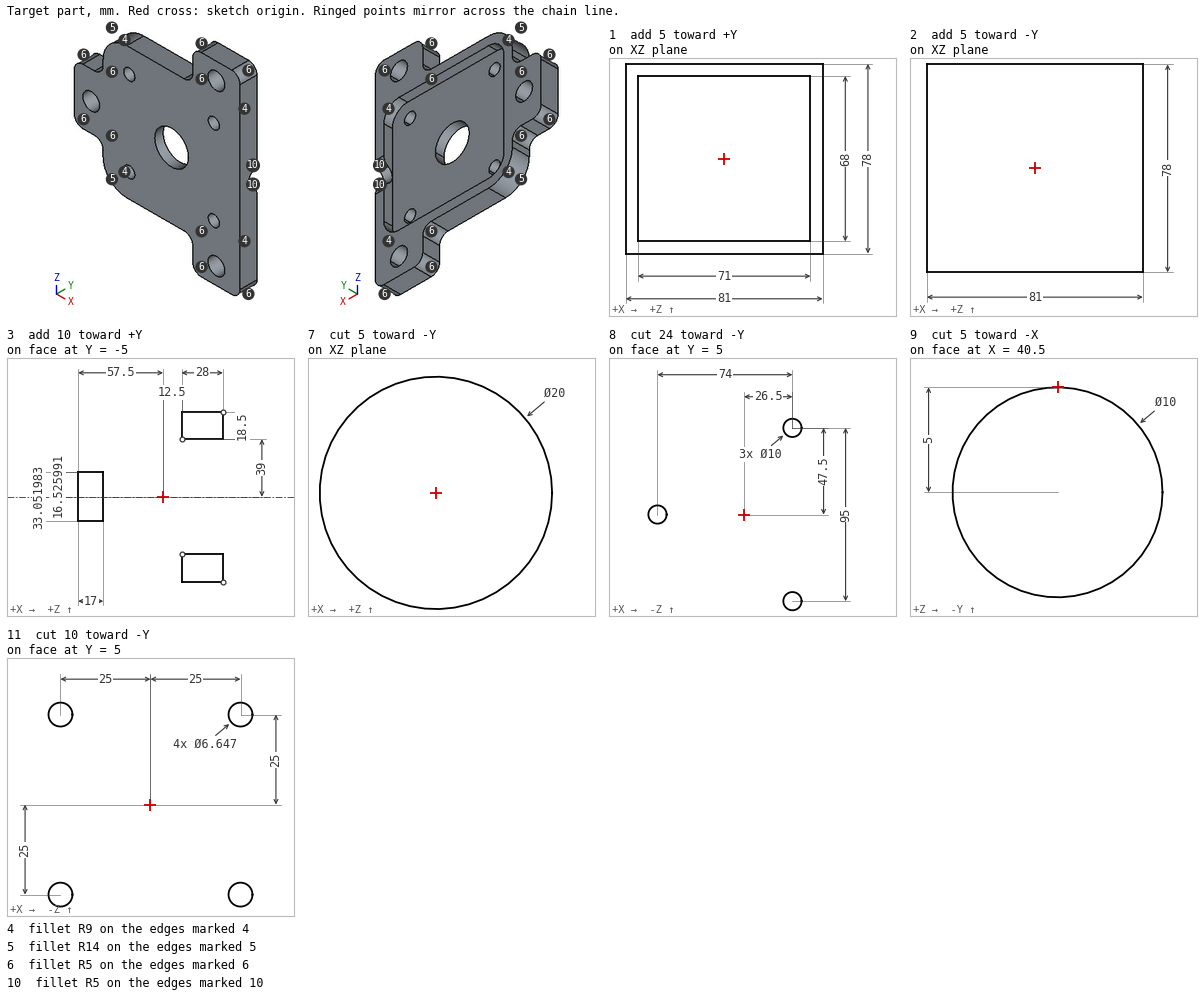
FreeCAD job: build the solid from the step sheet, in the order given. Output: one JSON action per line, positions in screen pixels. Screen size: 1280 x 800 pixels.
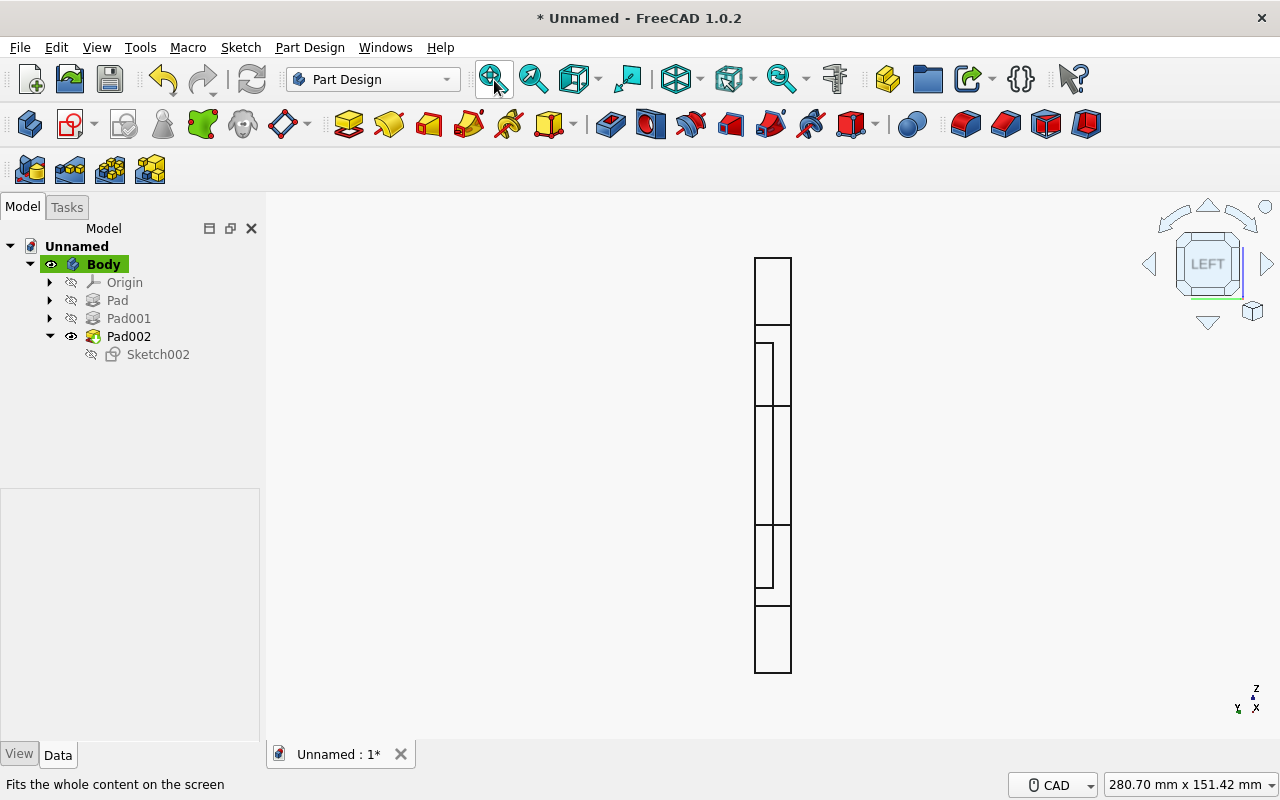
{"action": "key", "text": "0"}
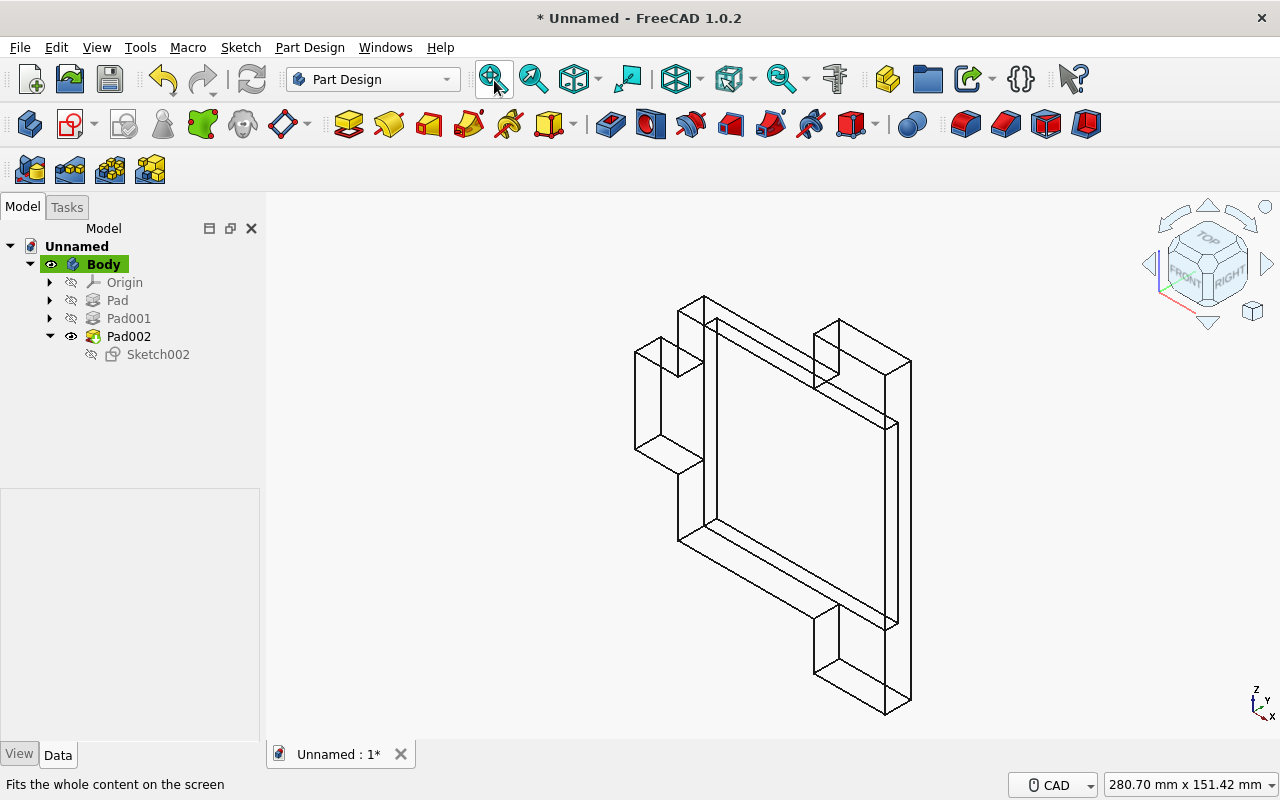
{"action": "left_click", "coordinate": [892, 425]}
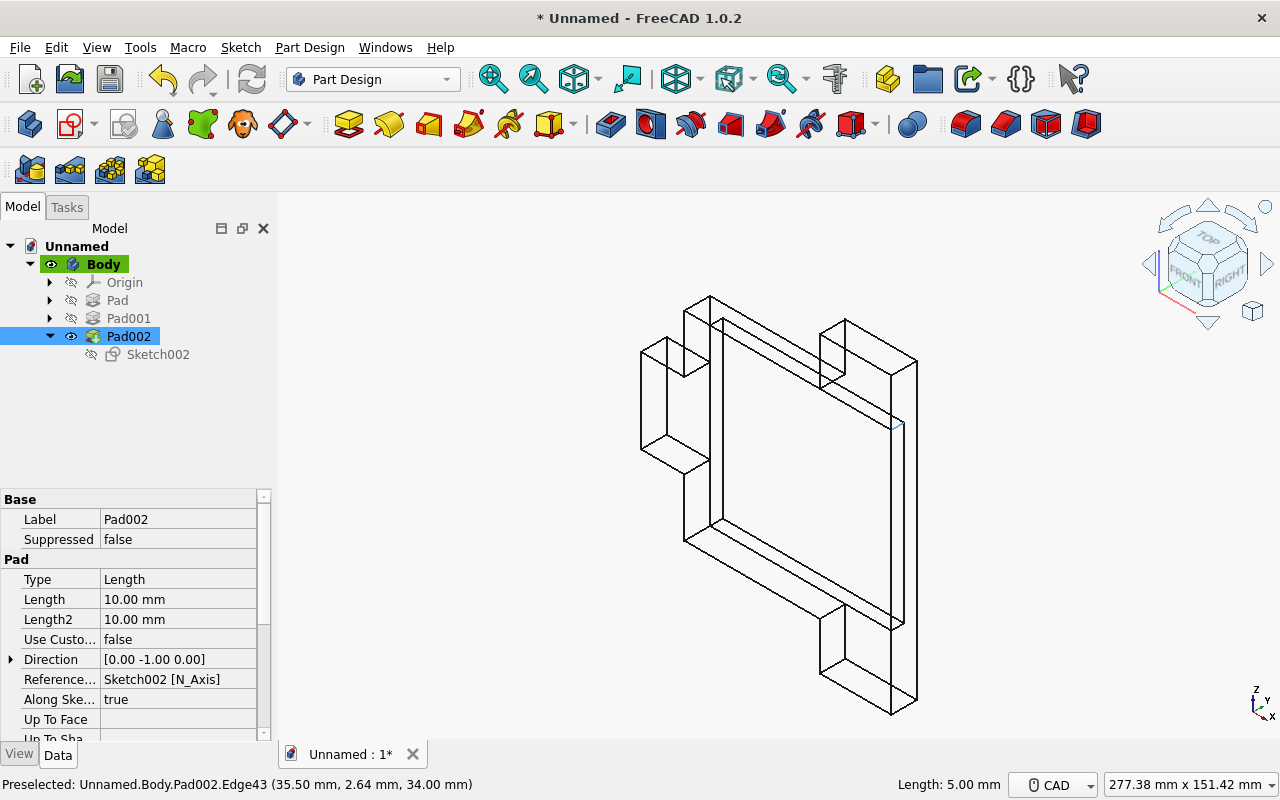
{"action": "left_click", "coordinate": [898, 626], "text": "ctrl"}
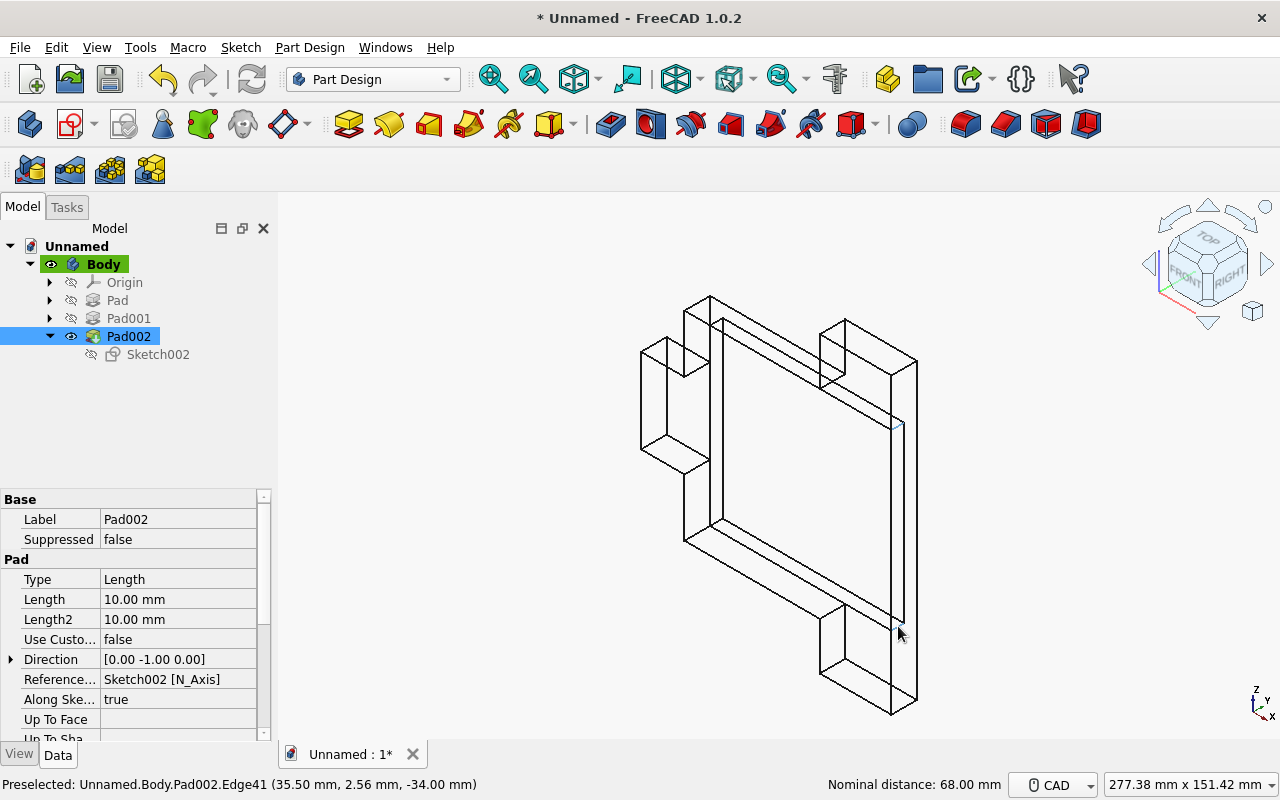
{"action": "left_click", "coordinate": [718, 521], "text": "ctrl"}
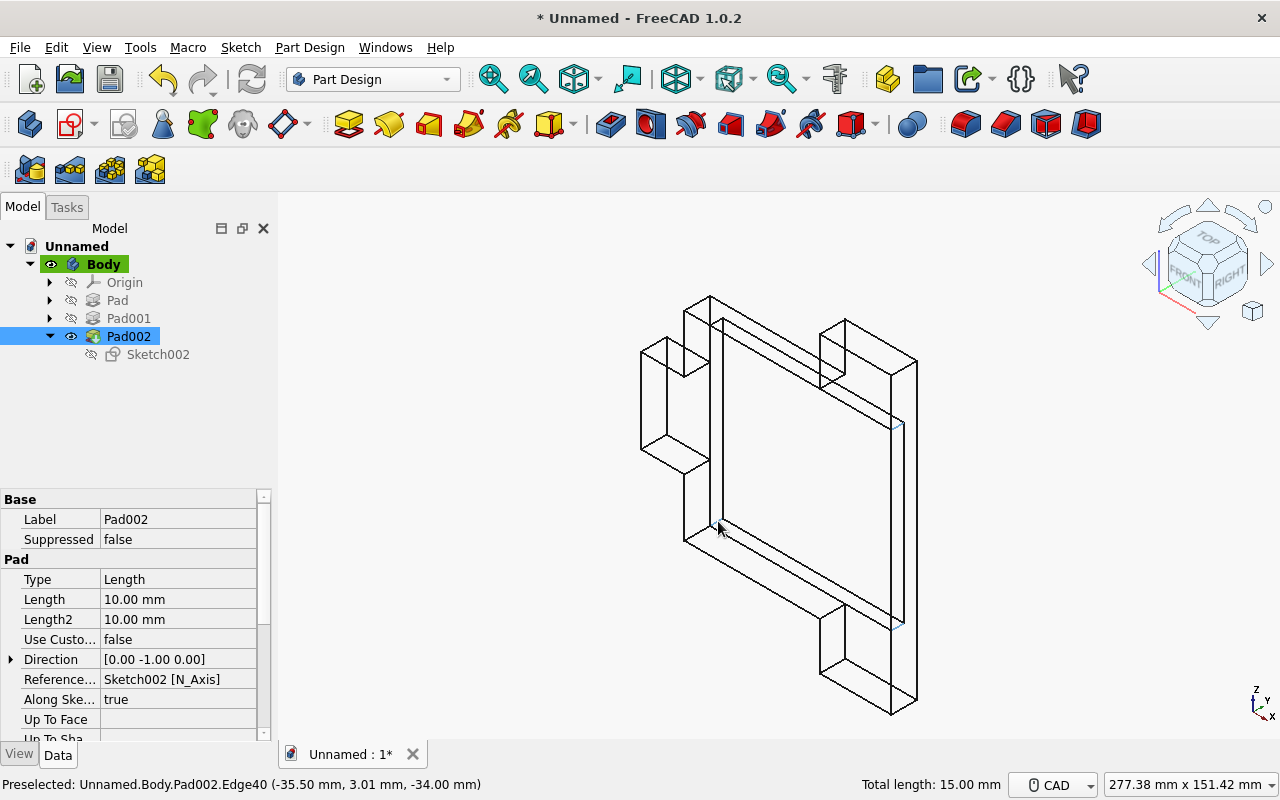
{"action": "left_click", "coordinate": [718, 320], "text": "ctrl"}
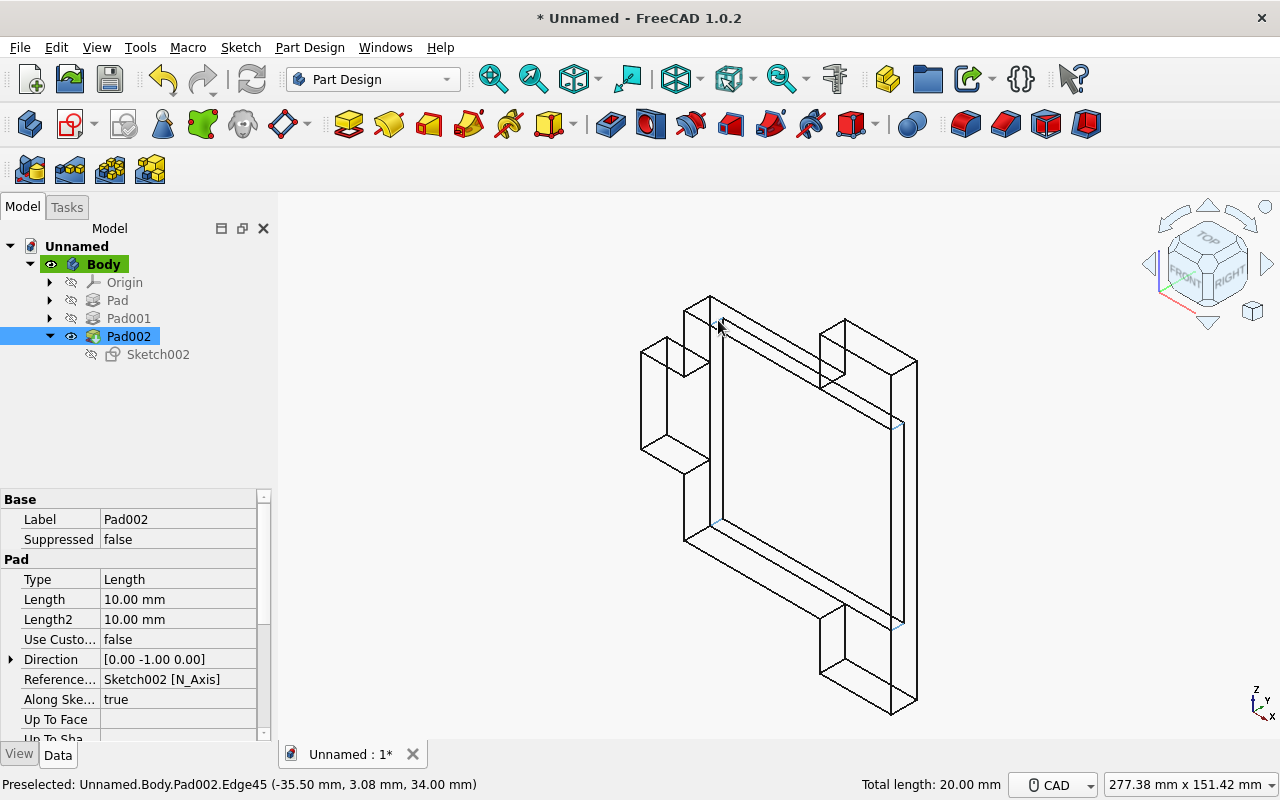
{"action": "key", "text": "v 1"}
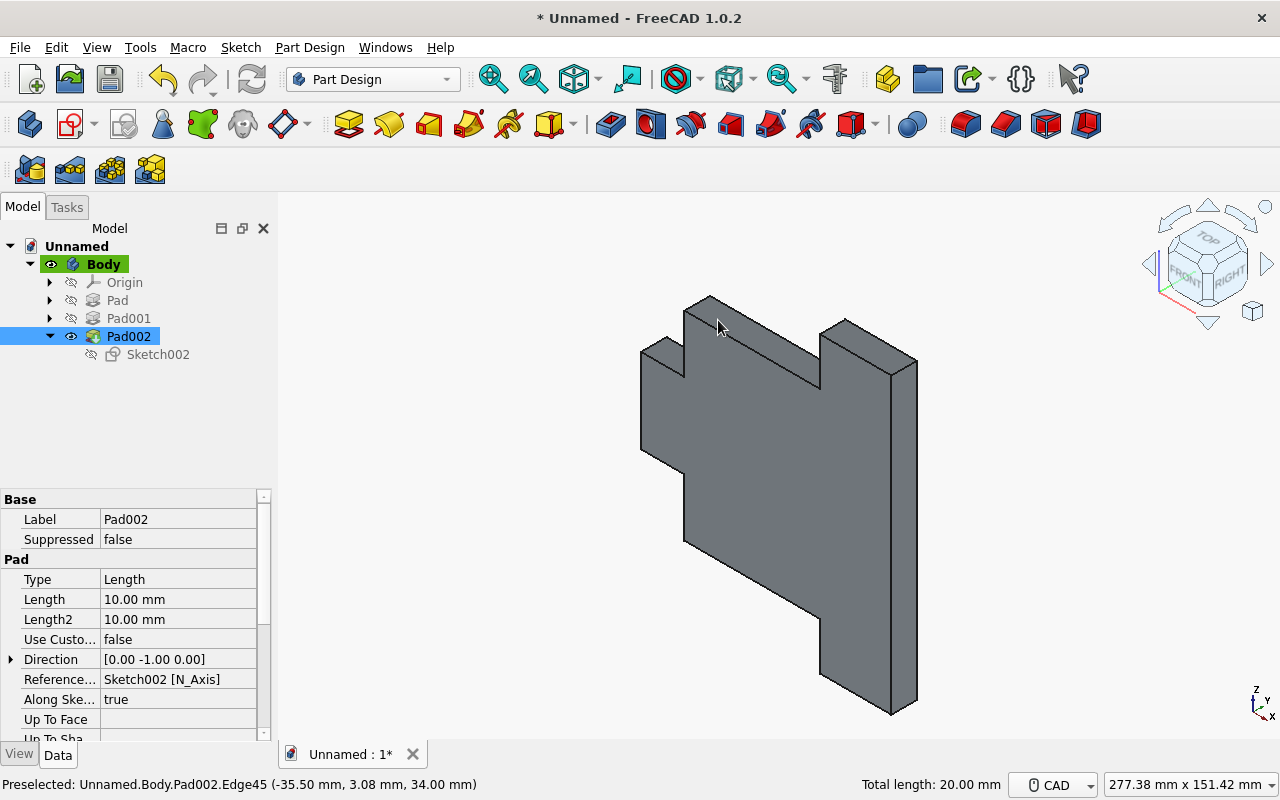
{"action": "left_click", "coordinate": [966, 124]}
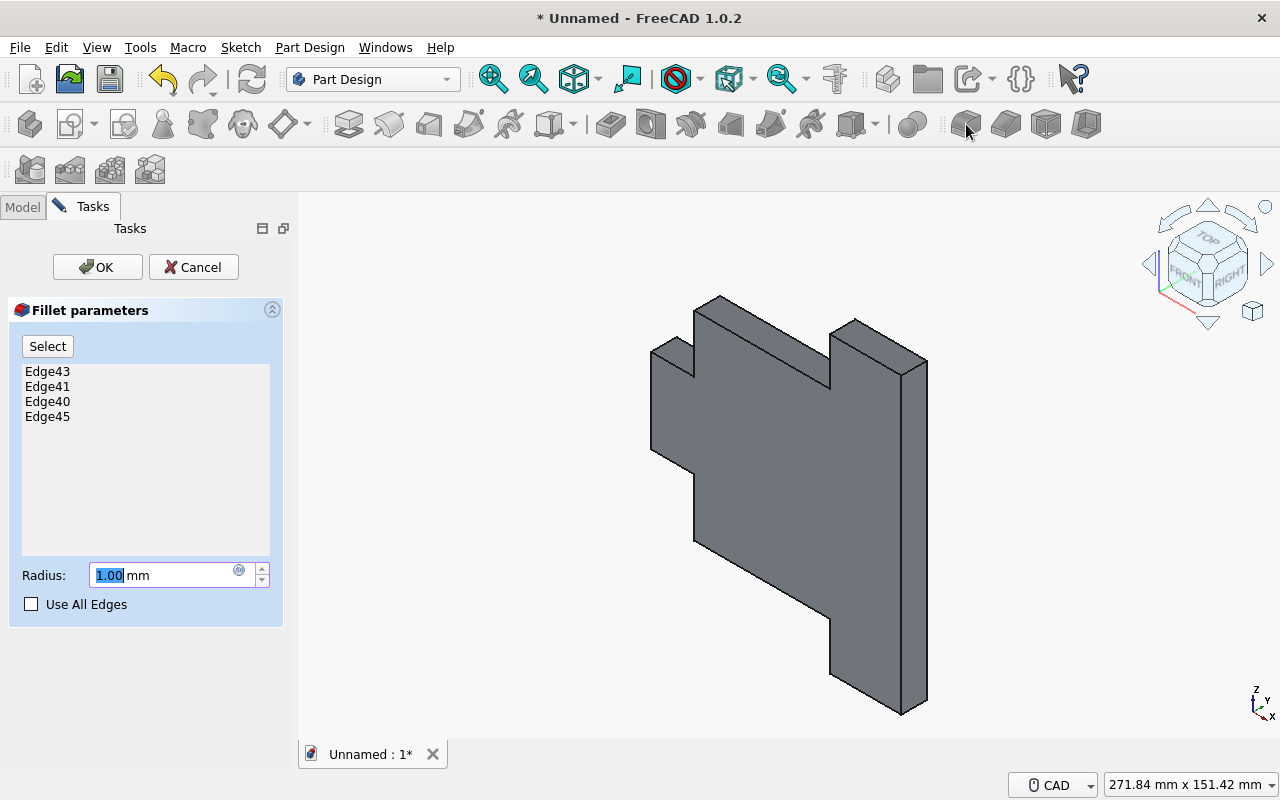
{"action": "type", "text": "9"}
{"action": "key", "text": "Tab"}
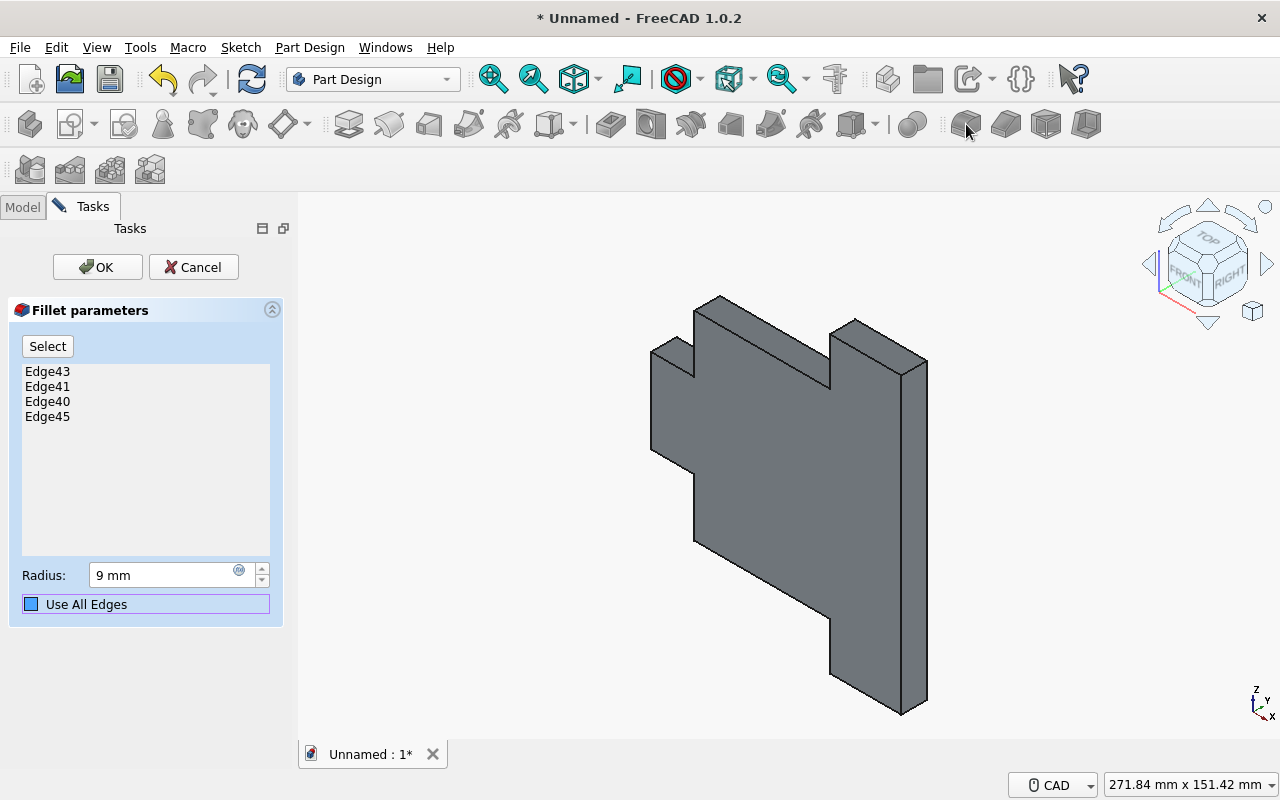
{"action": "left_click", "coordinate": [98, 267]}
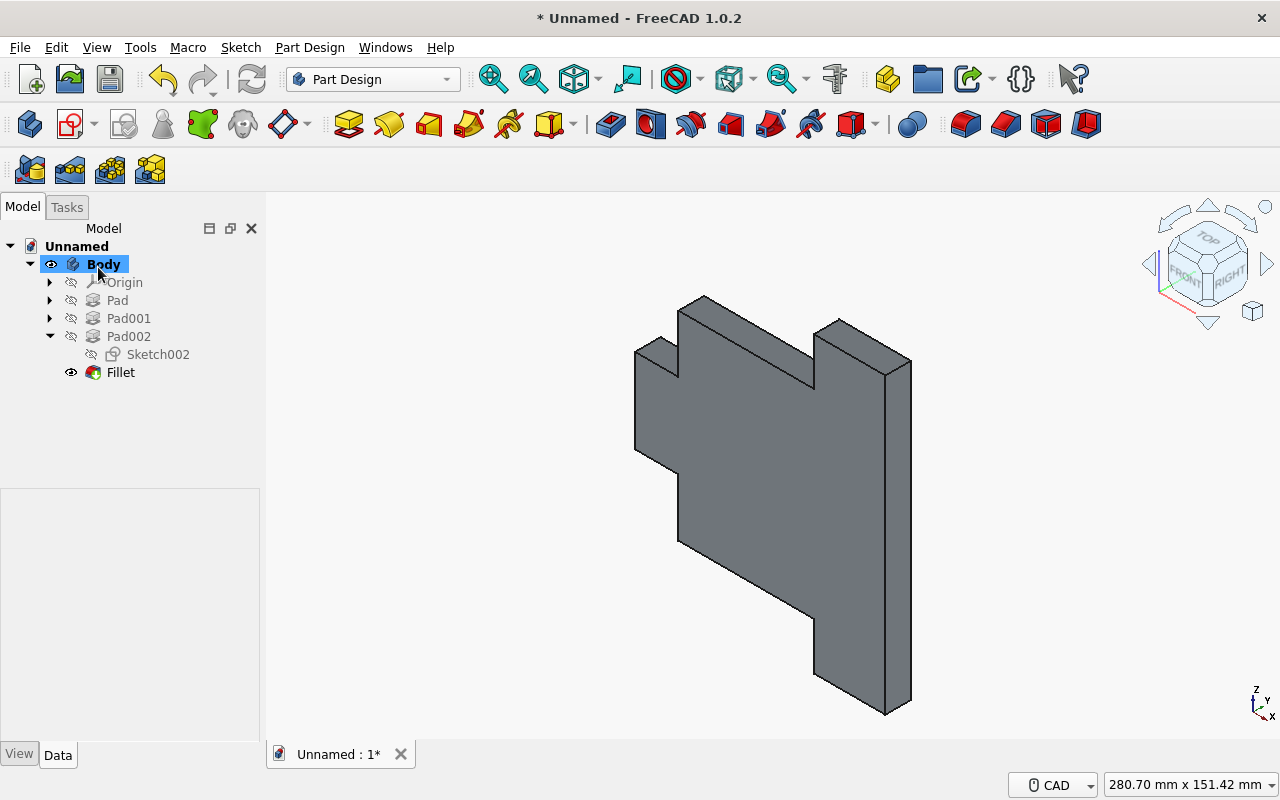
{"action": "key", "text": "2"}